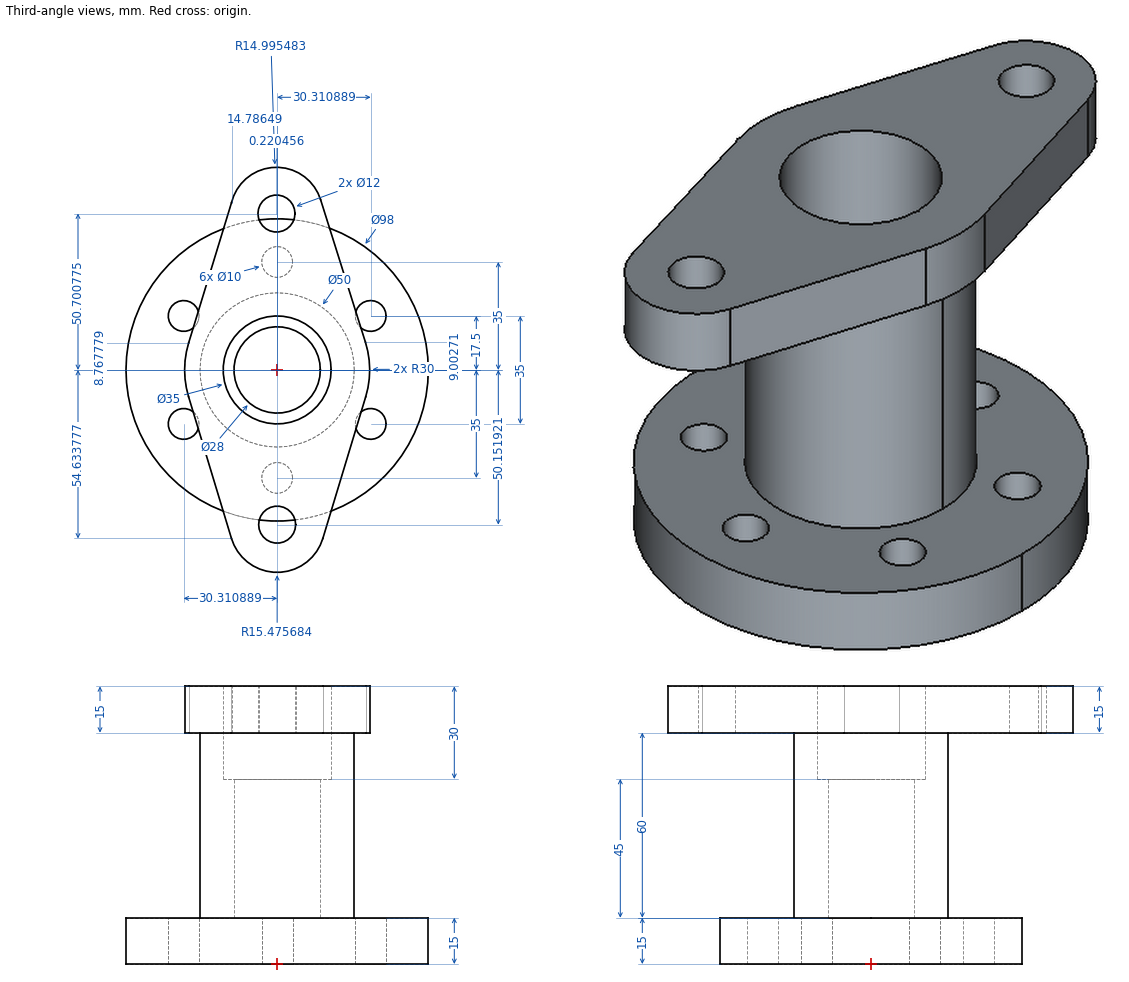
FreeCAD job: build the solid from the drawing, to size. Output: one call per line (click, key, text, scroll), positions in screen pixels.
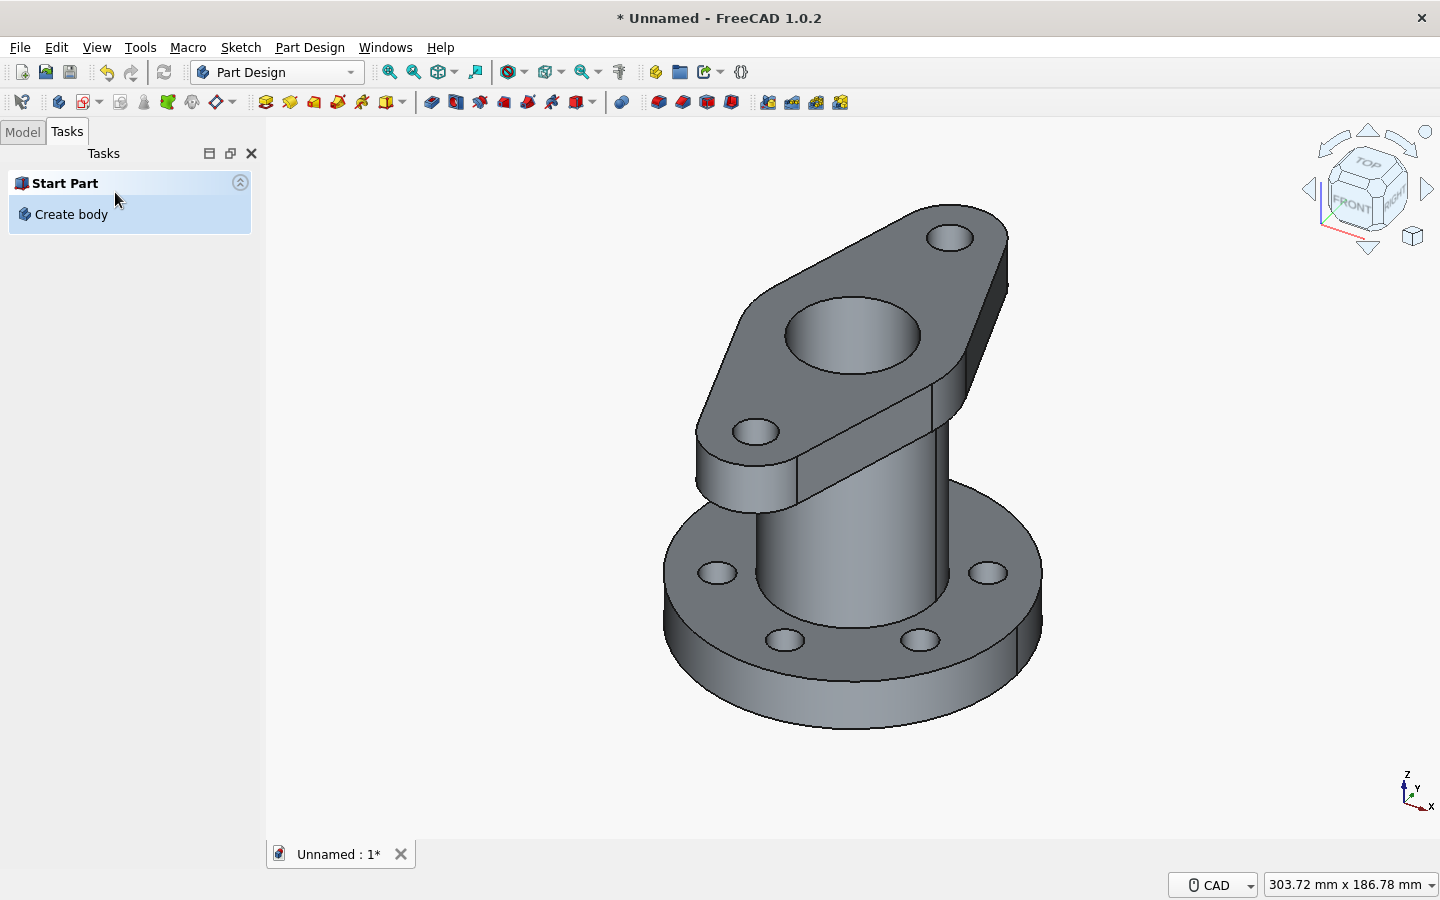
key(0)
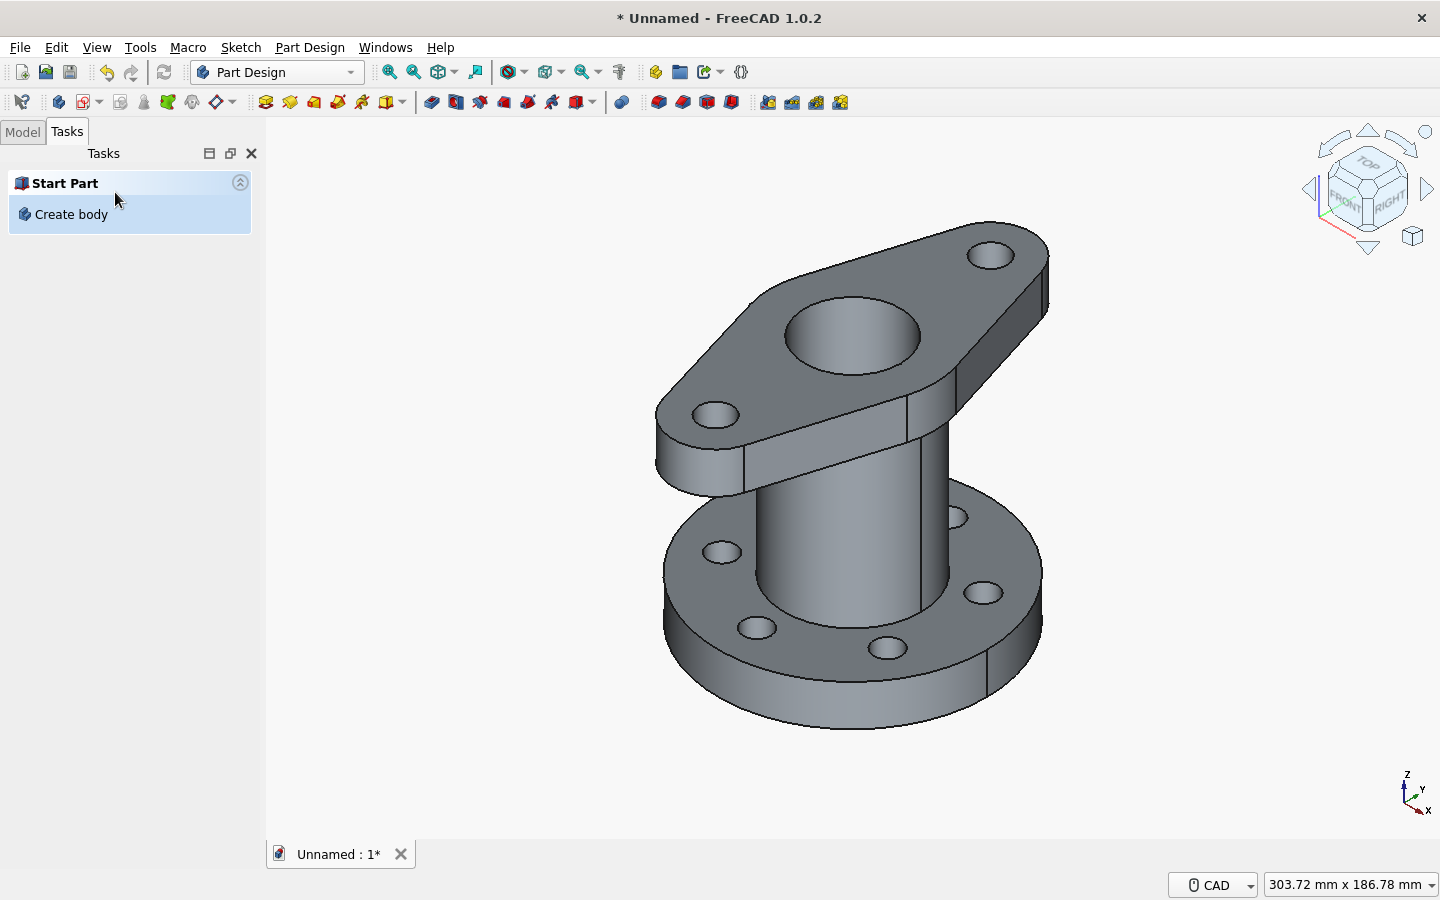
key(2)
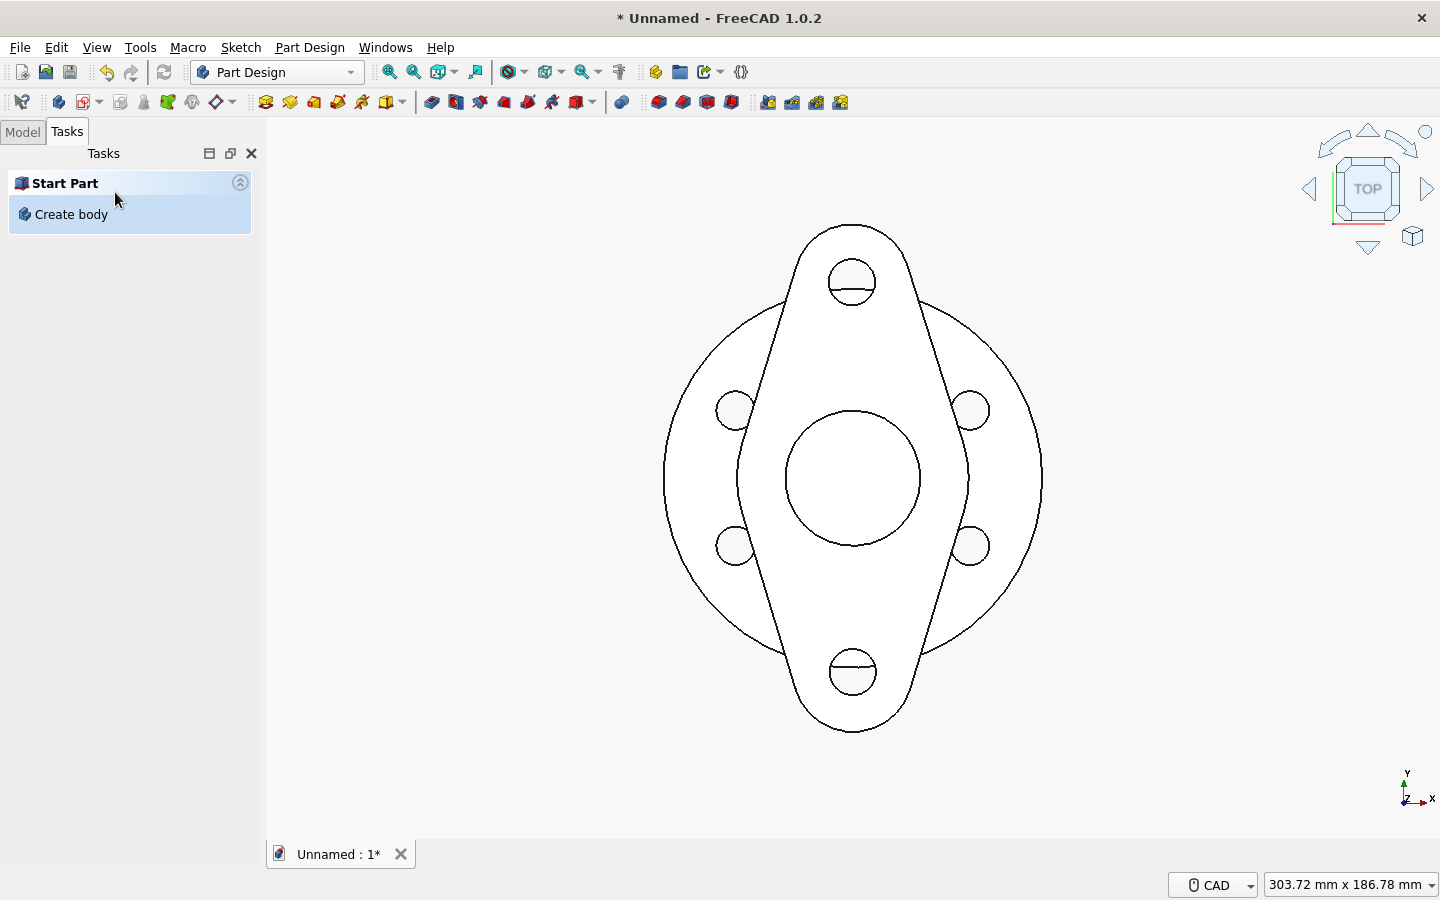
click(853, 477)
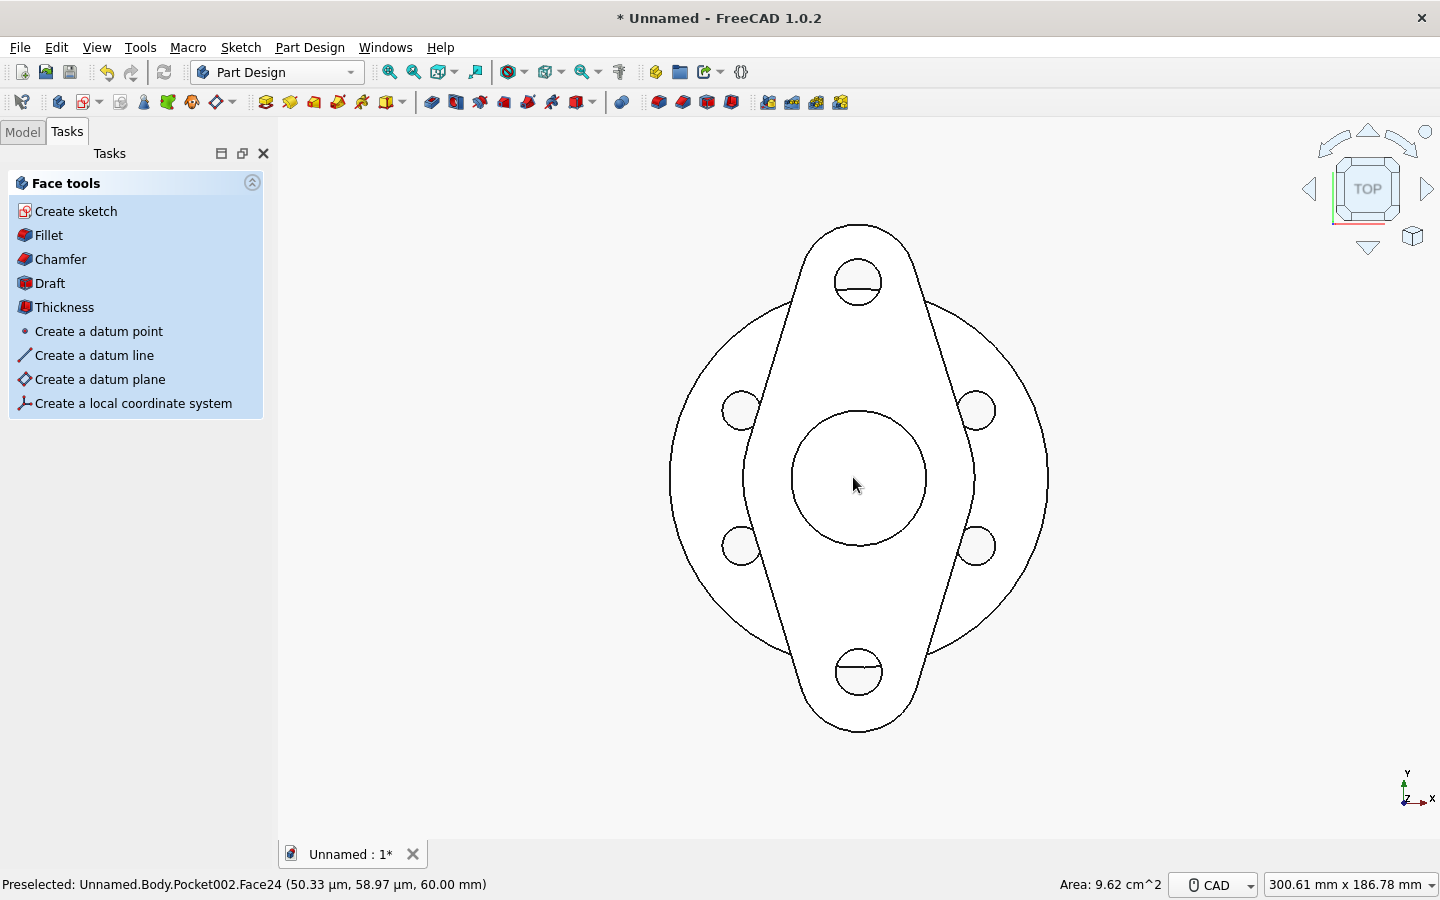
click(84, 102)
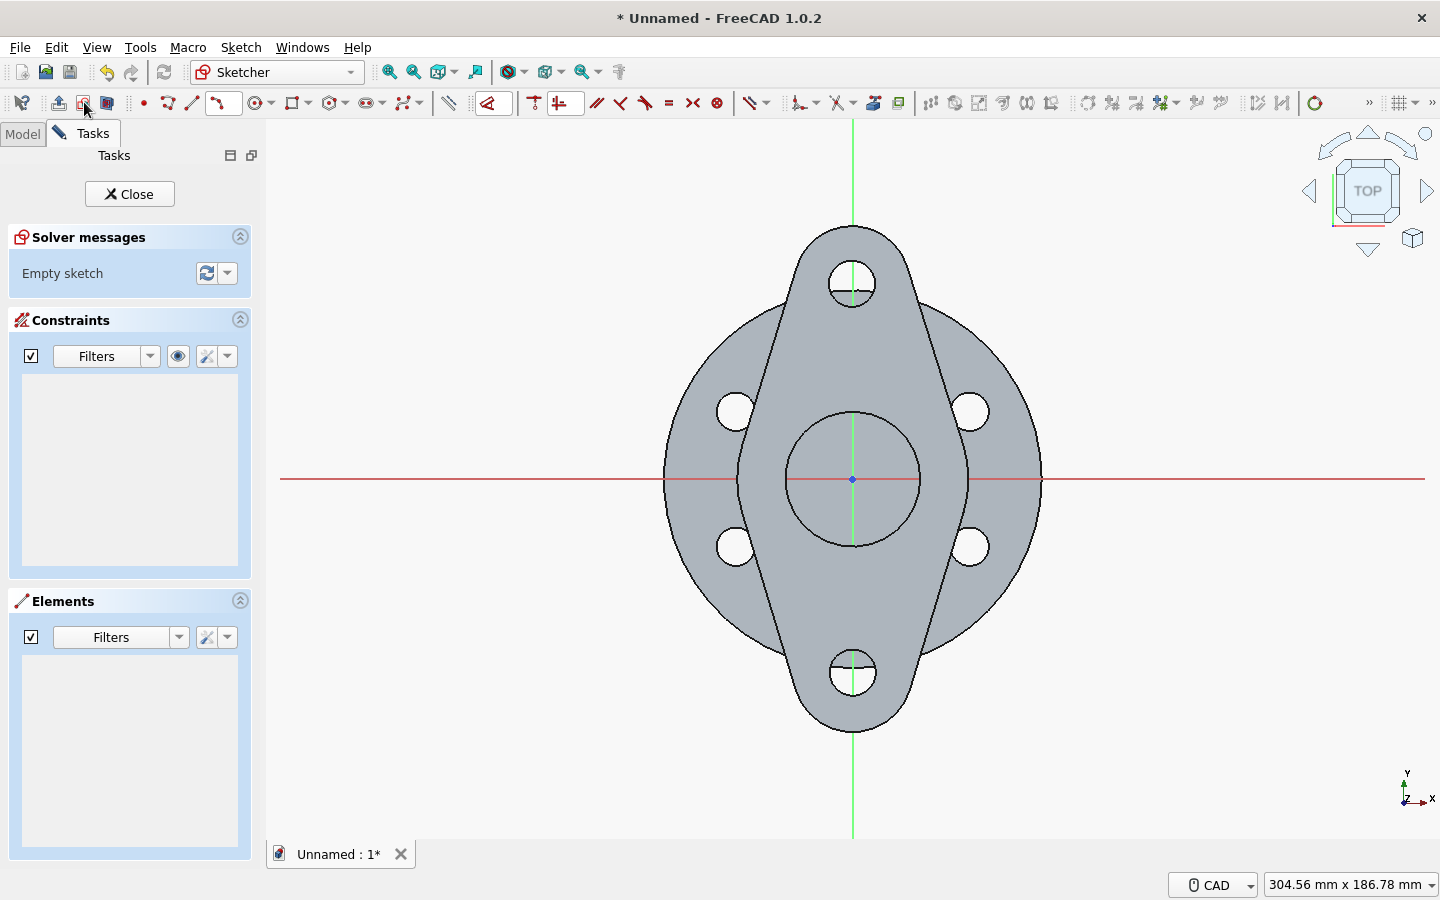
scroll(875, 479, up, 7)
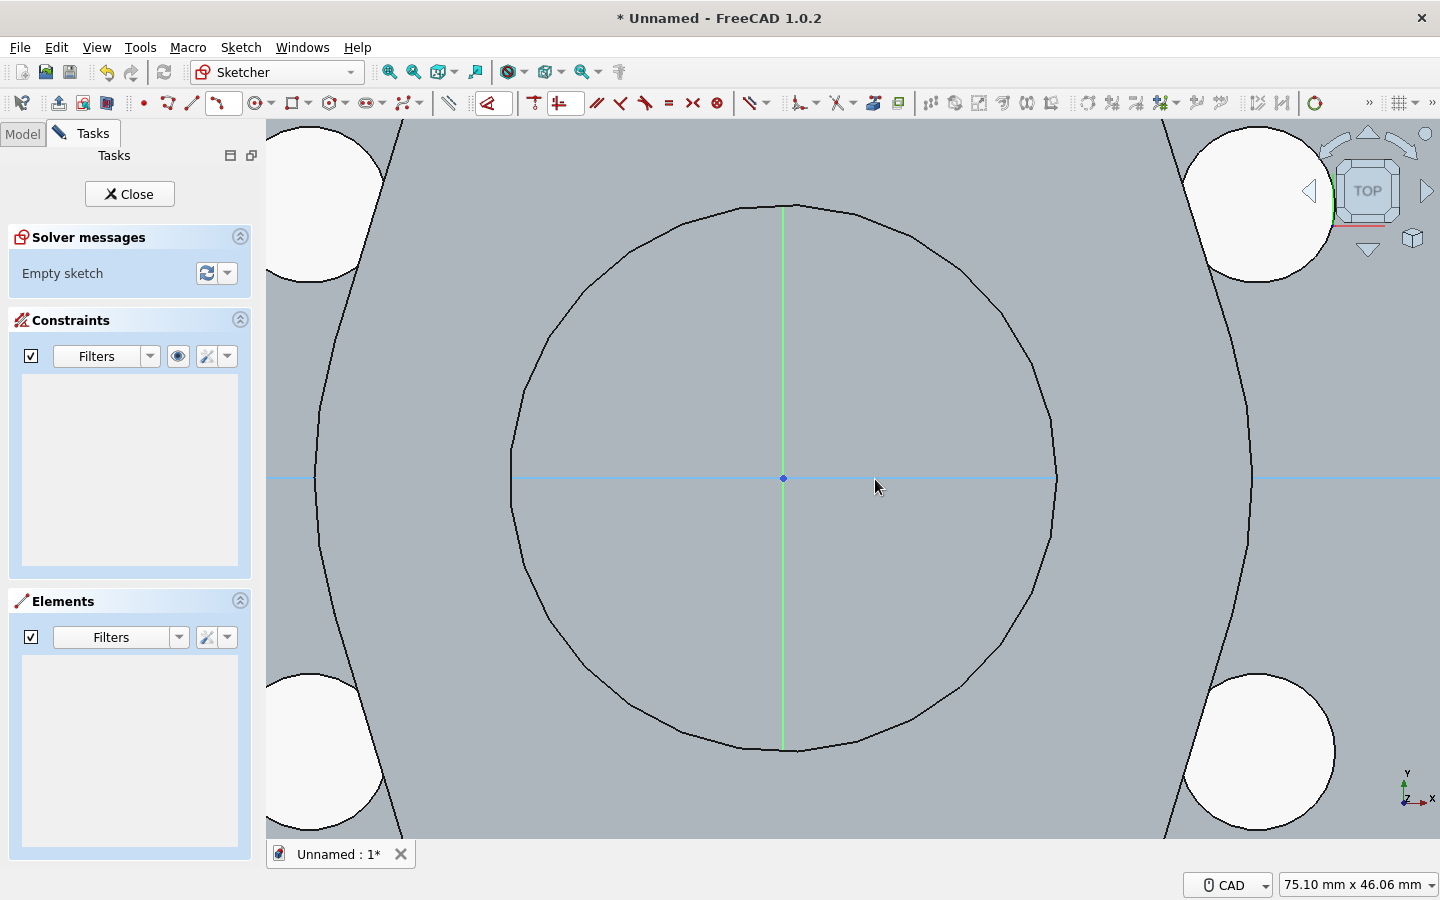
key(g)
key(c)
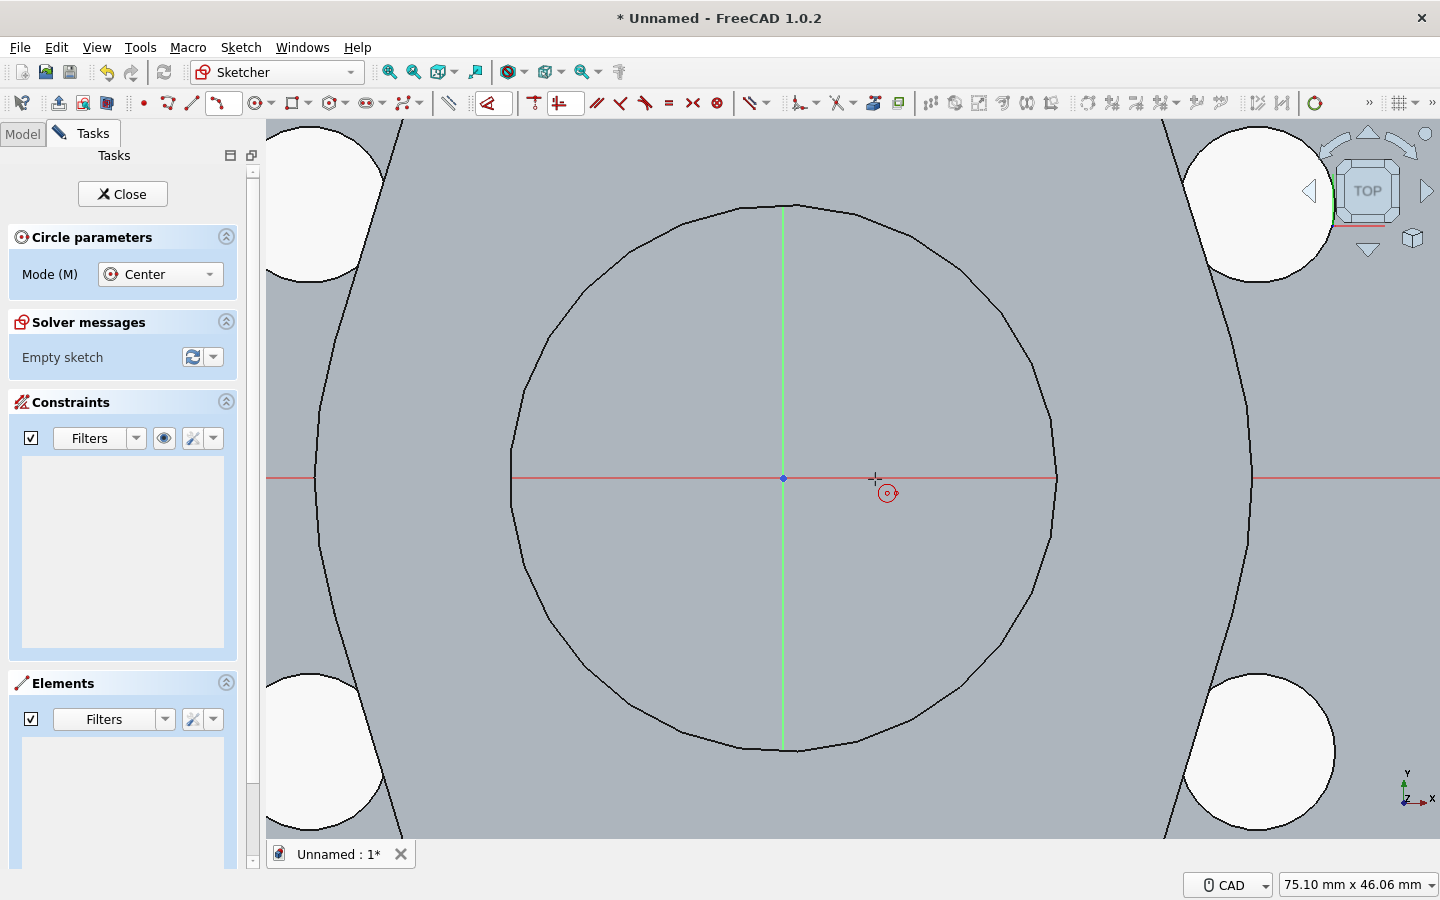
click(783, 478)
click(938, 324)
key(Escape)